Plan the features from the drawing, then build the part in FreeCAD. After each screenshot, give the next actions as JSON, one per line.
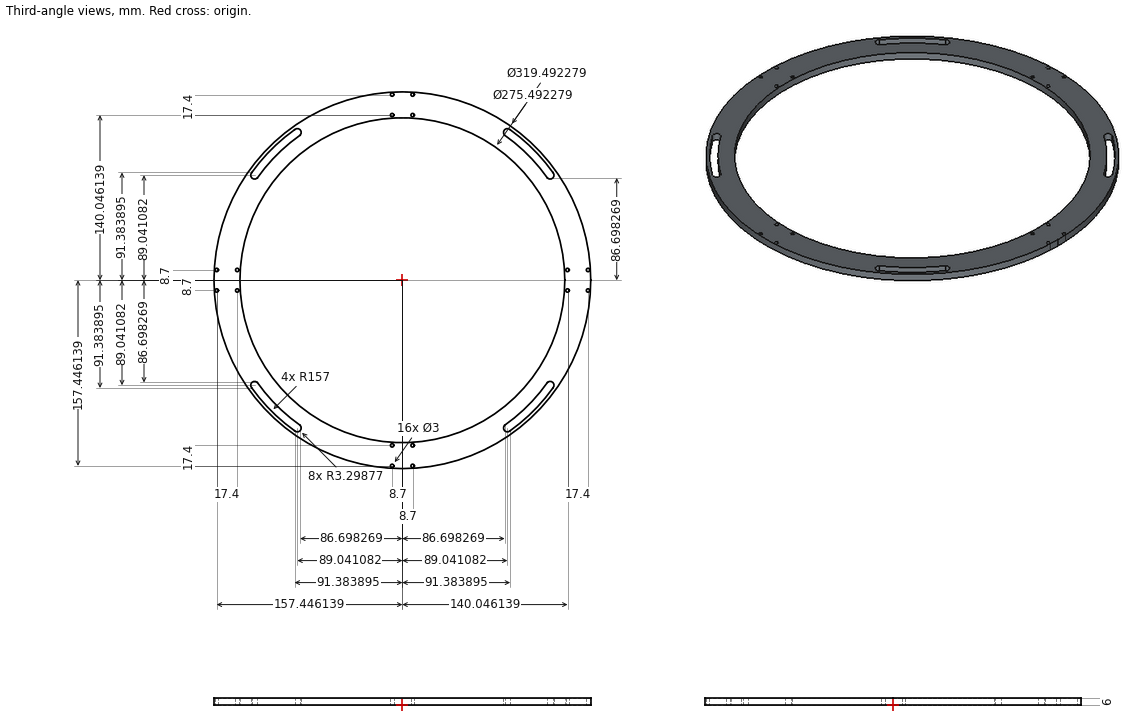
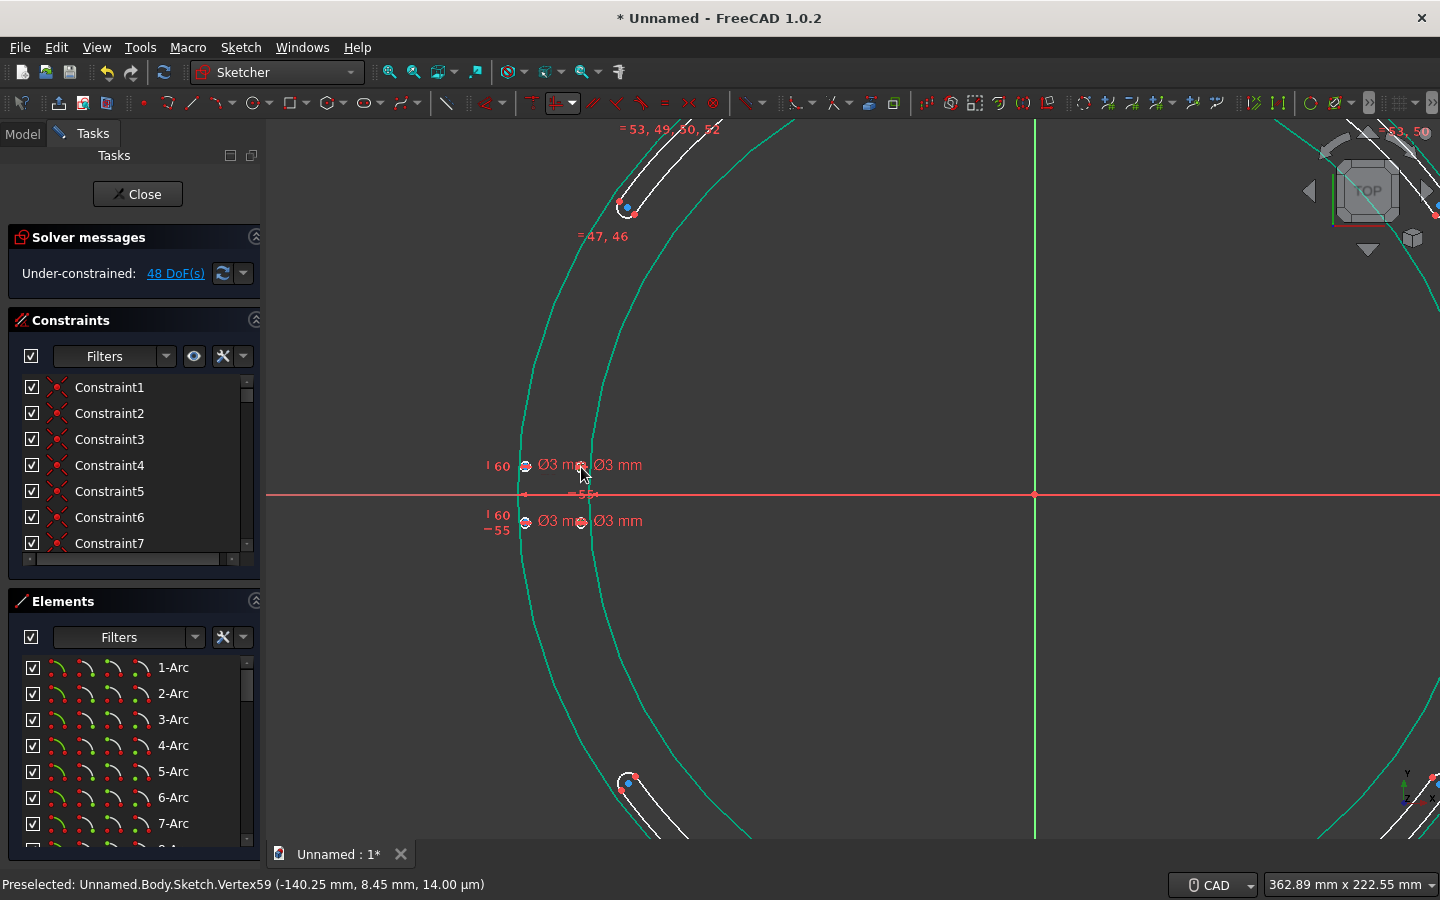
{"action": "key", "text": "v"}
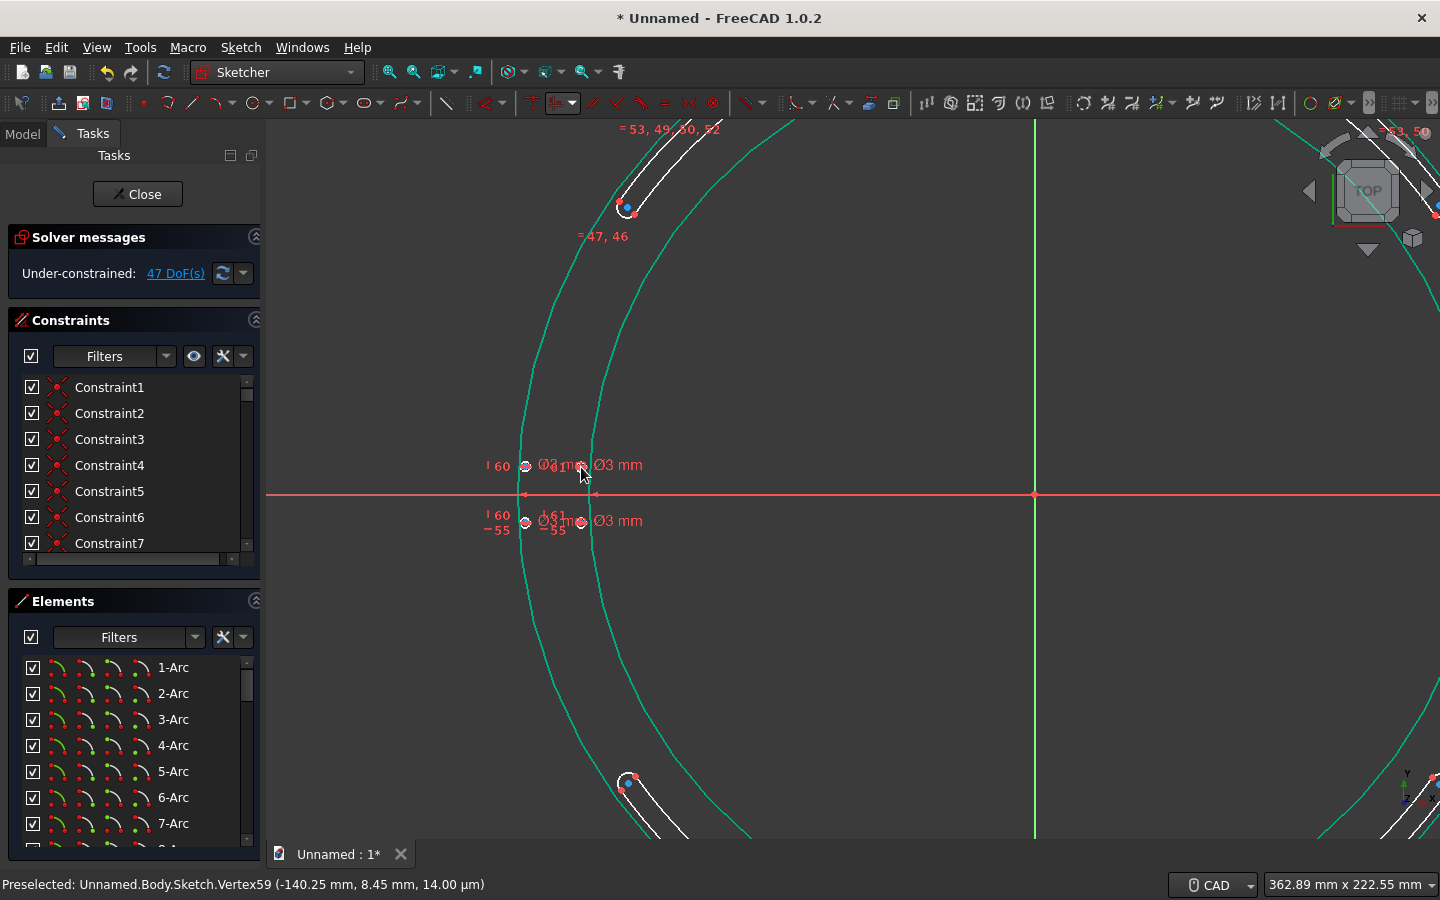
{"action": "left_click", "coordinate": [525, 467]}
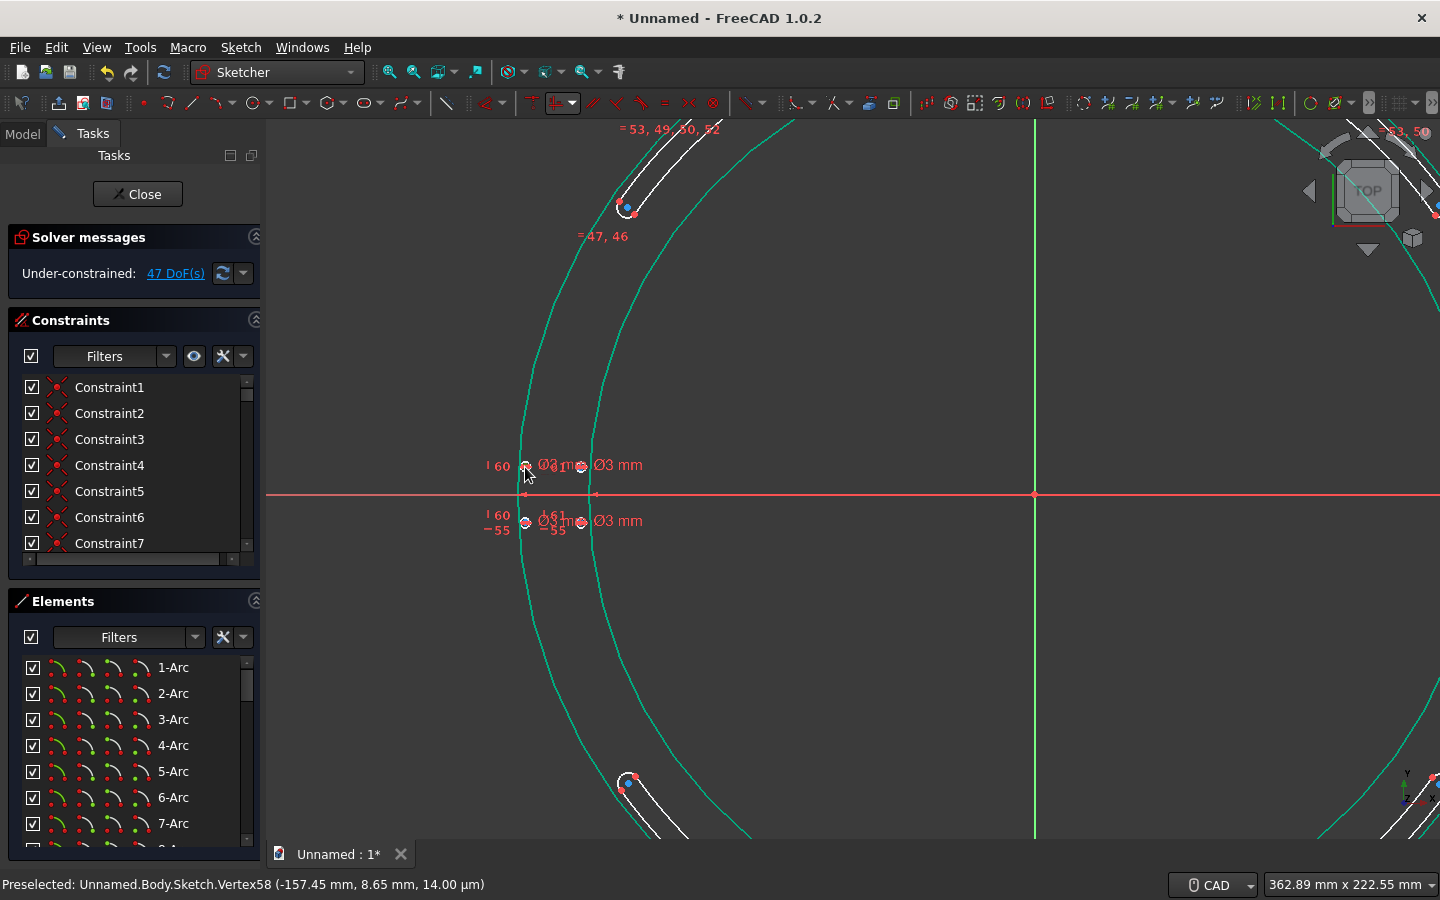
{"action": "left_click", "coordinate": [581, 467]}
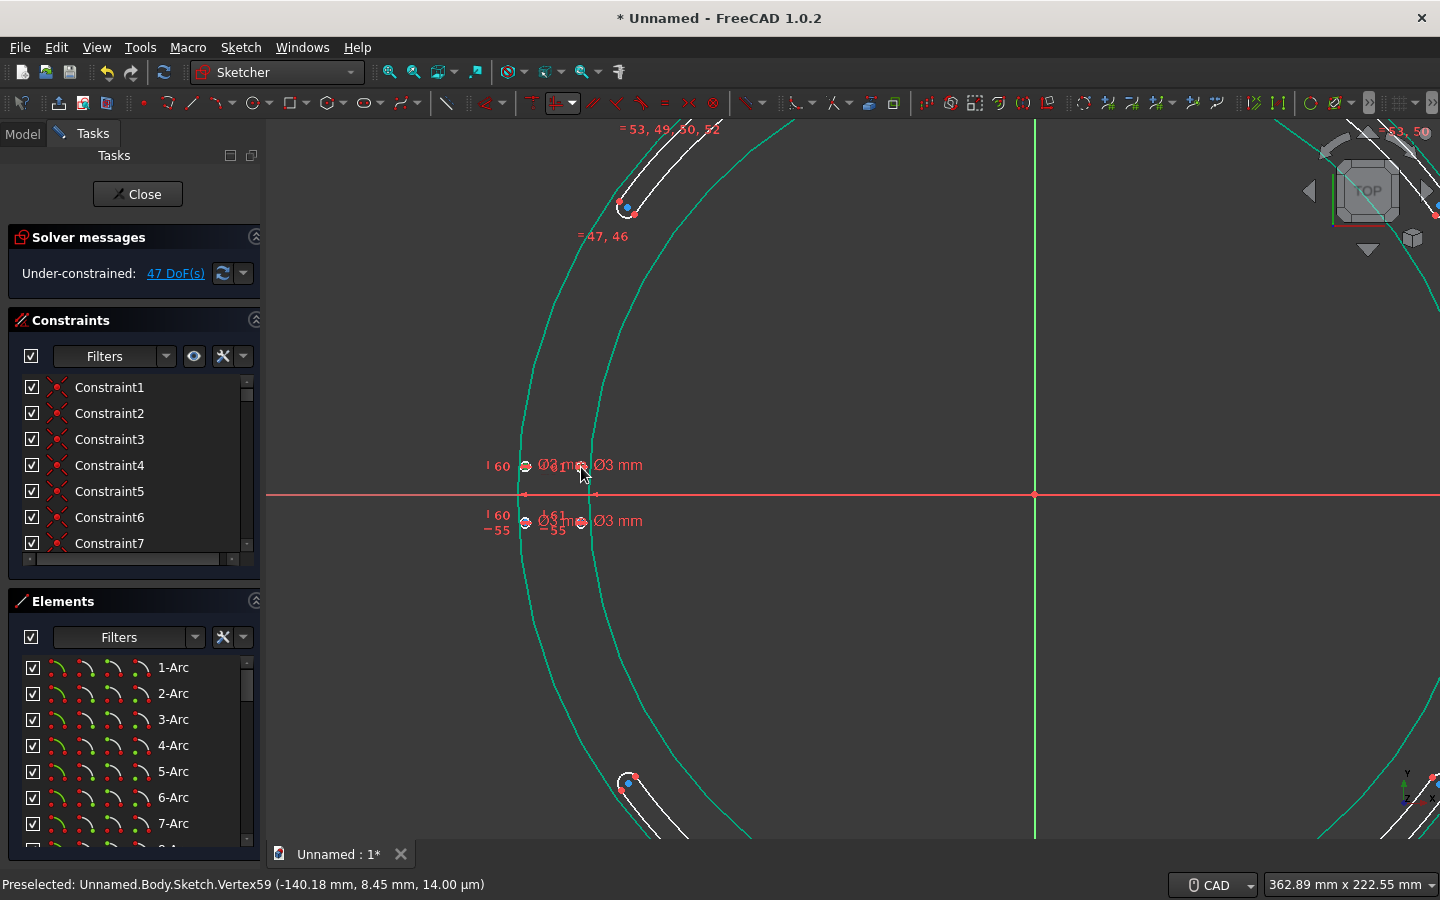
{"action": "key", "text": "h"}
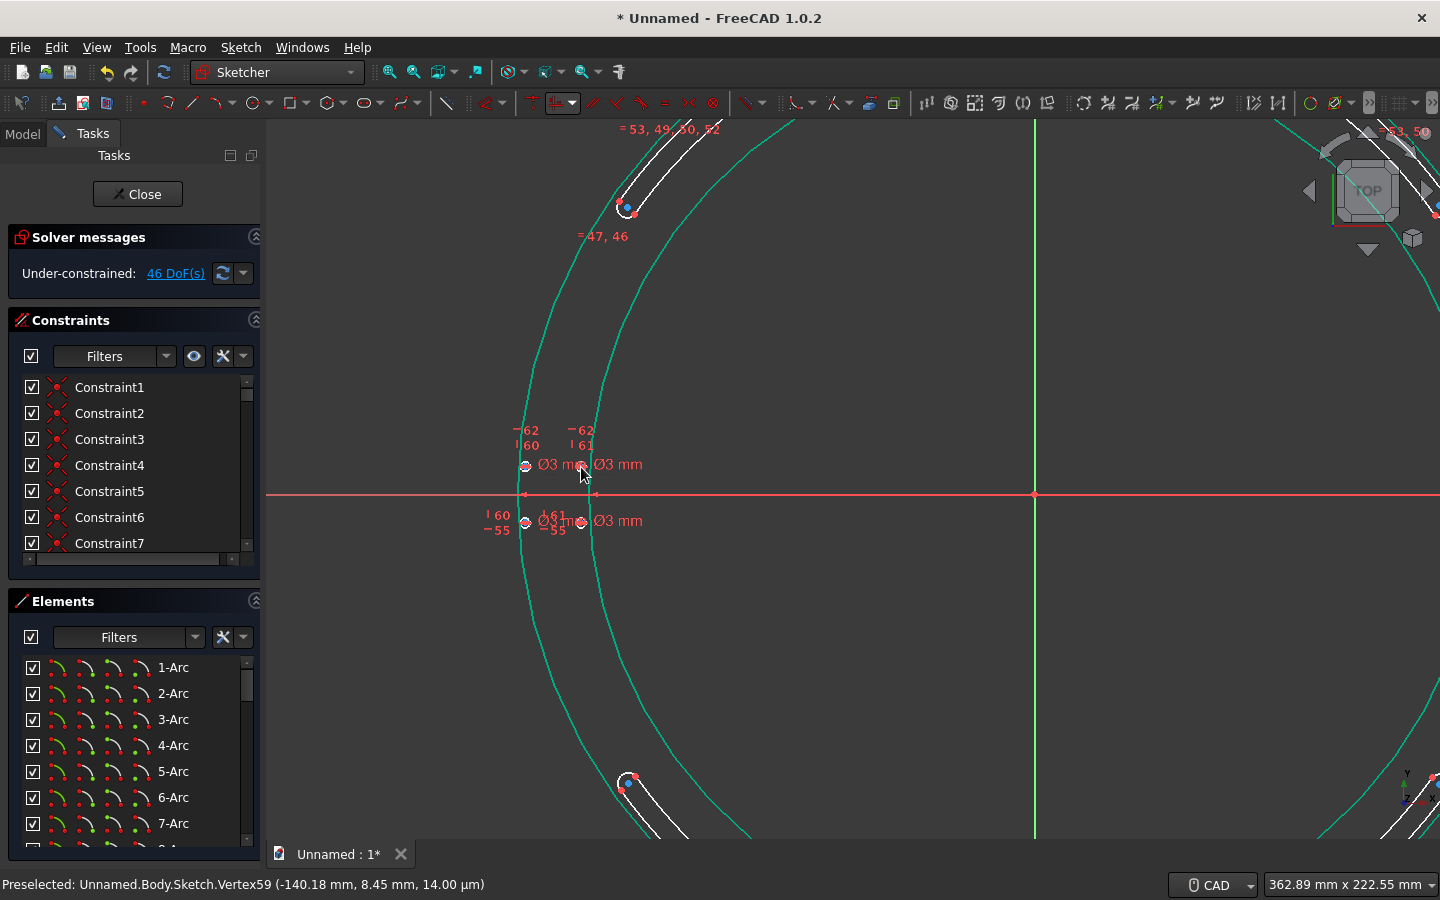
{"action": "scroll", "coordinate": [580, 466], "scroll_direction": "down", "scroll_amount": 4}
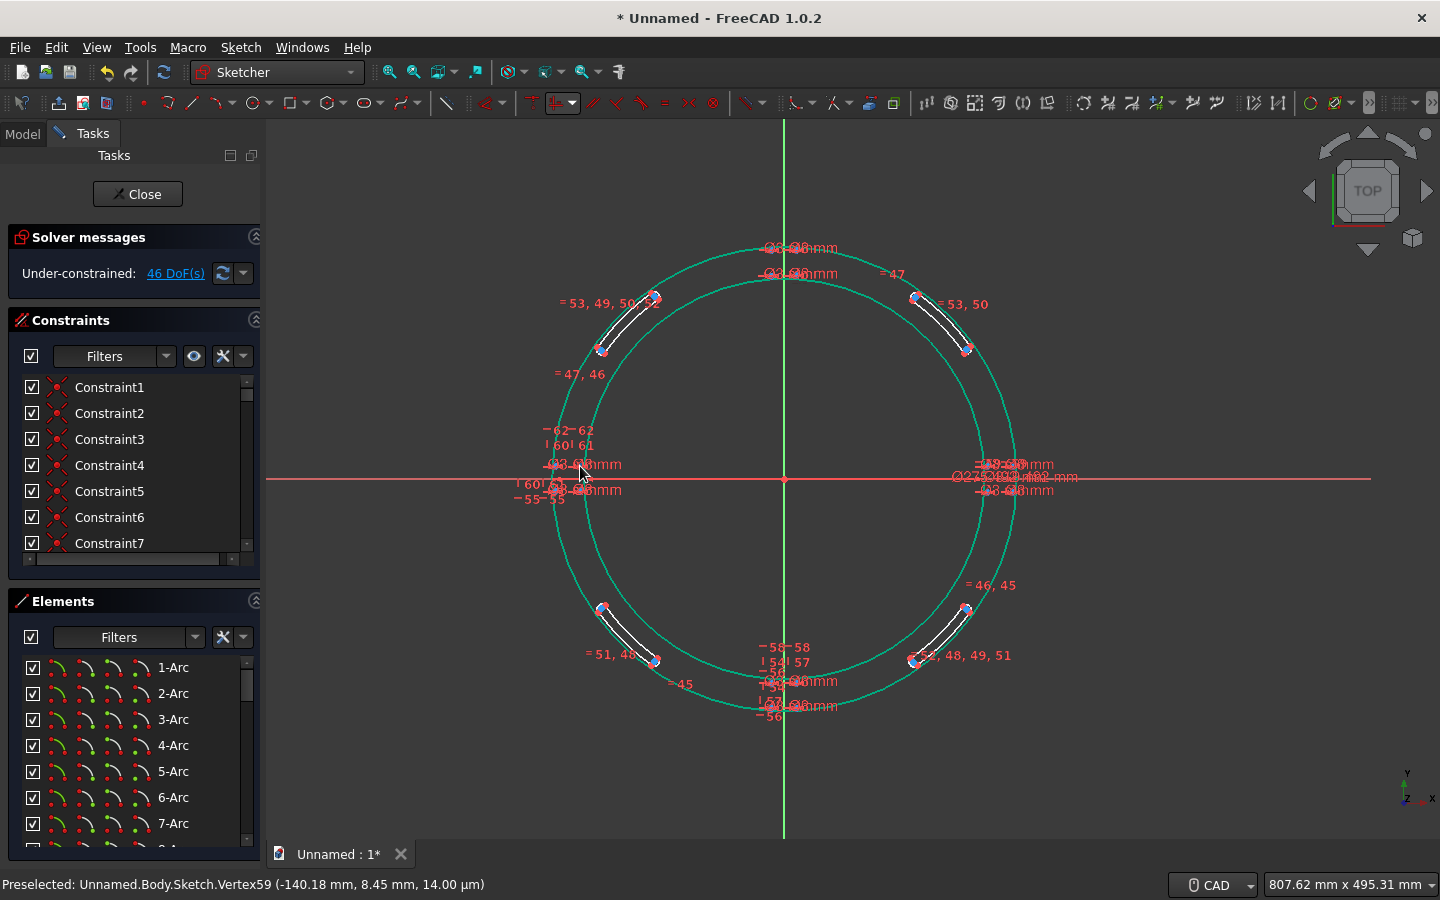
{"action": "left_click", "coordinate": [772, 276]}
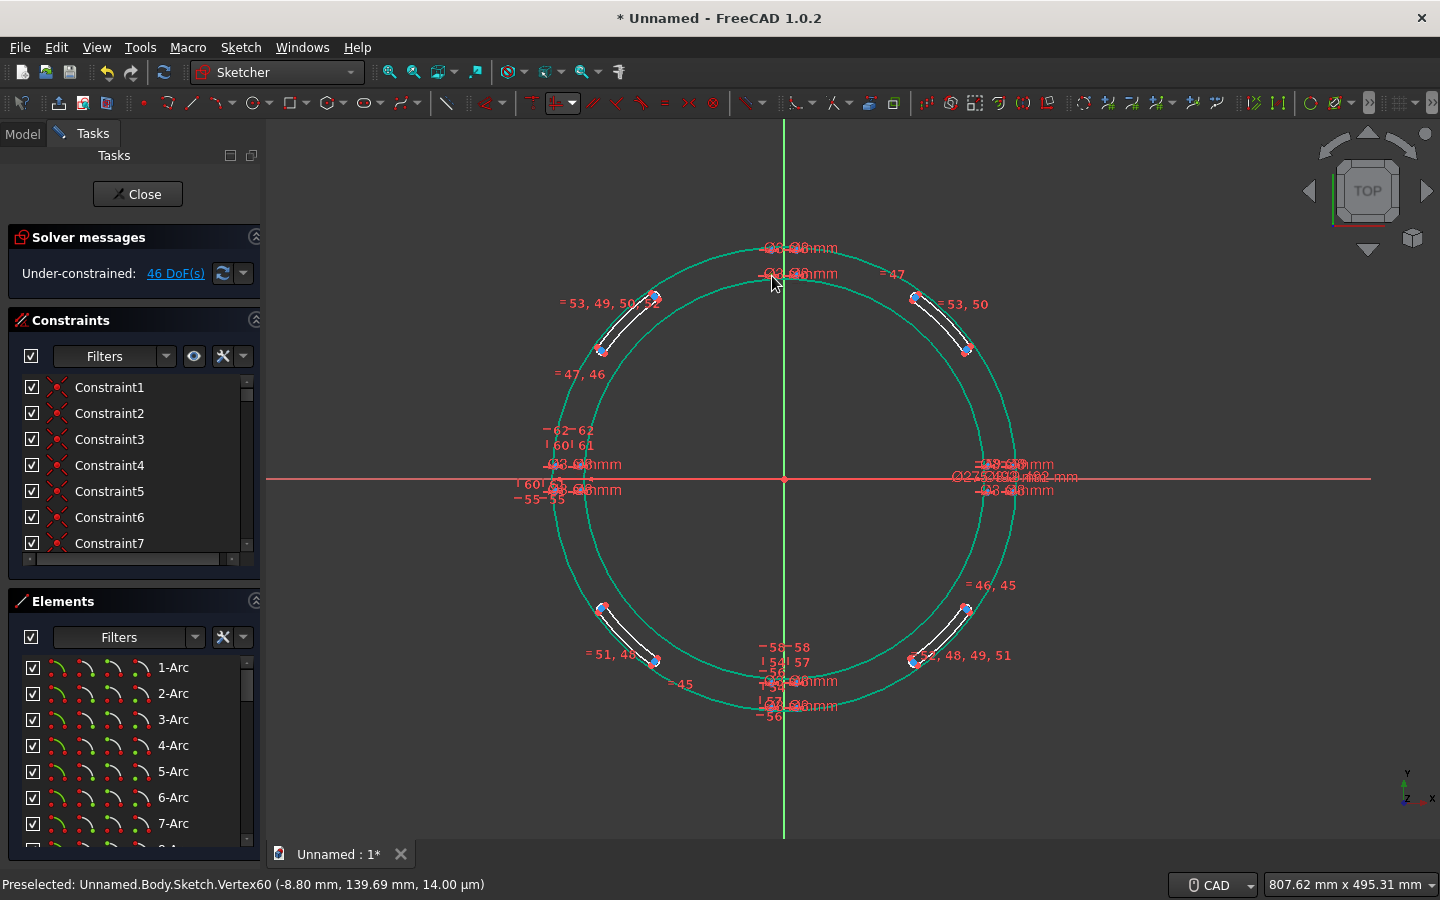
{"action": "left_click", "coordinate": [772, 250]}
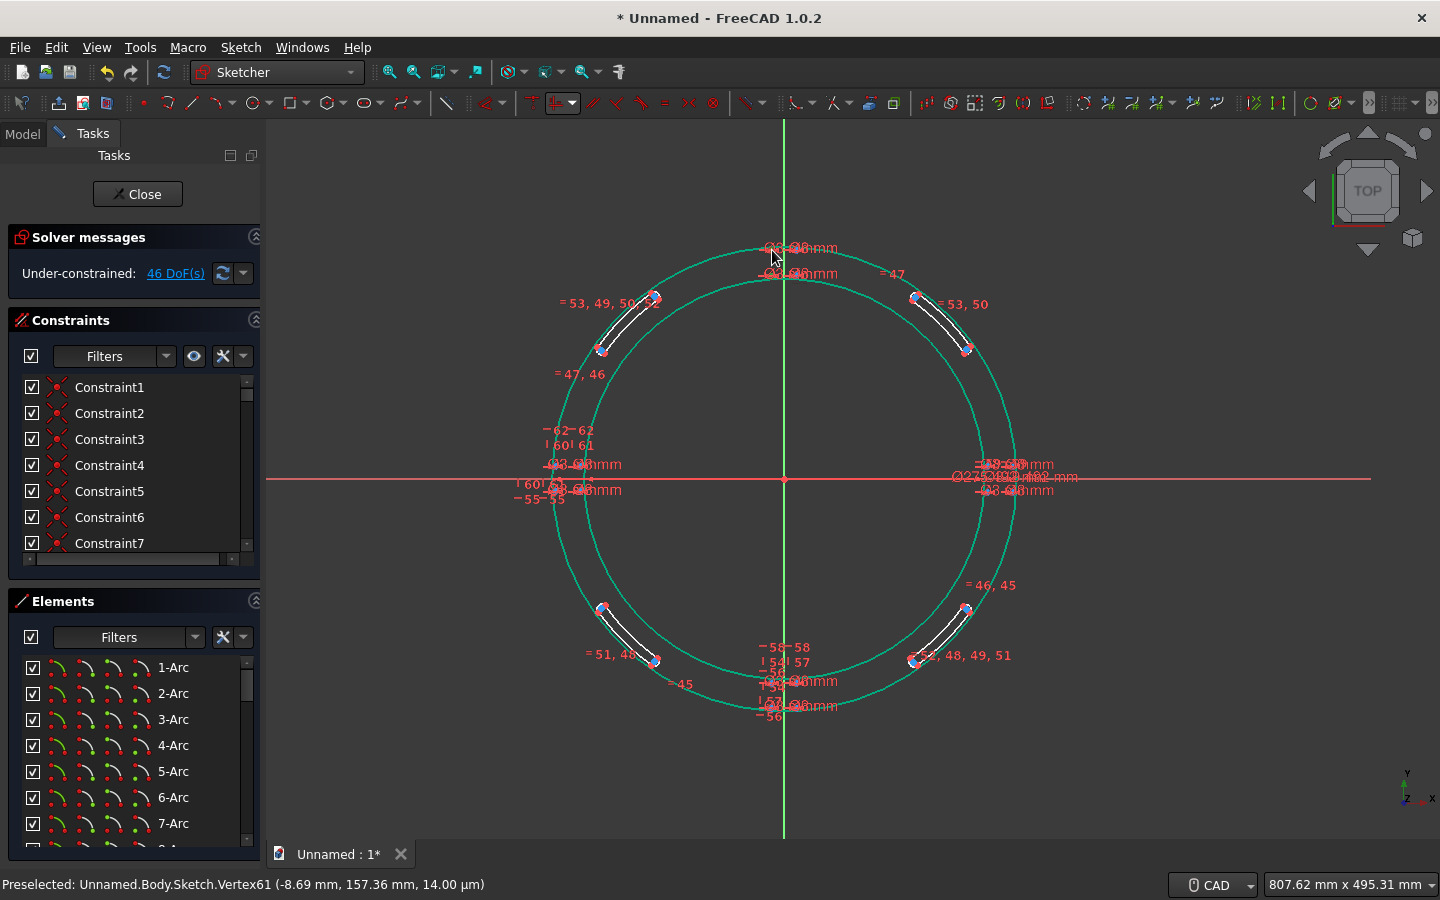
{"action": "key", "text": "v"}